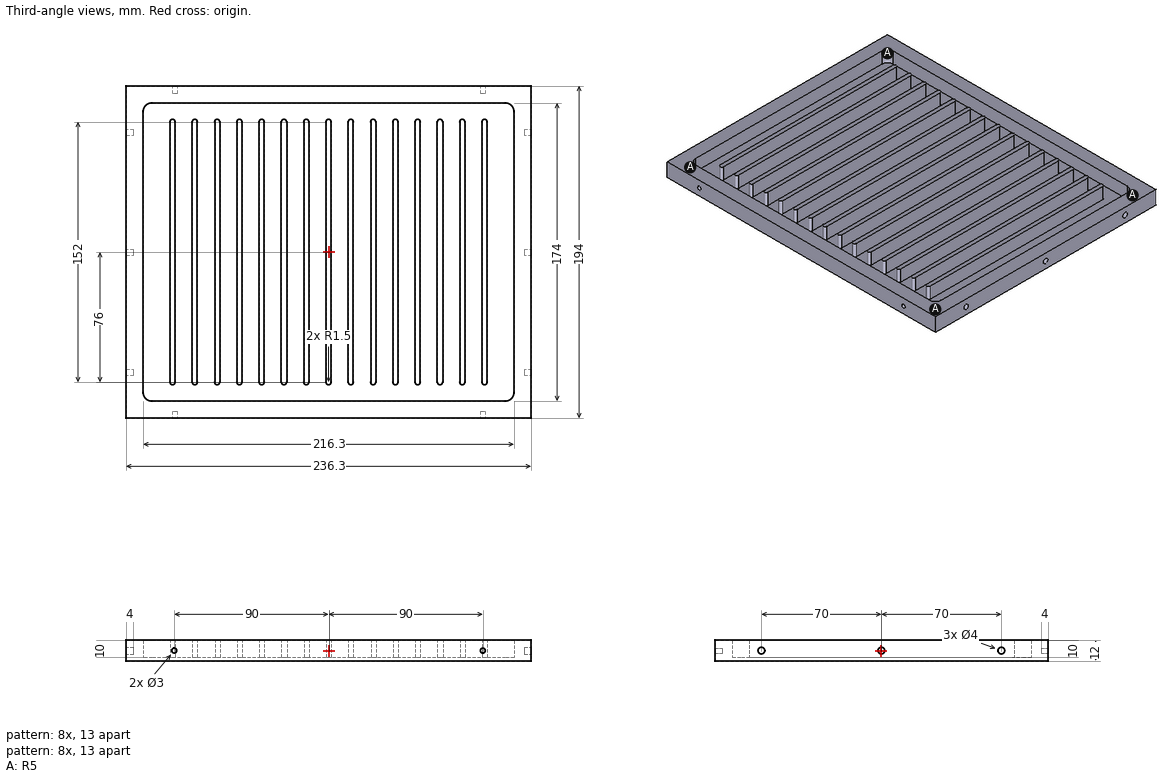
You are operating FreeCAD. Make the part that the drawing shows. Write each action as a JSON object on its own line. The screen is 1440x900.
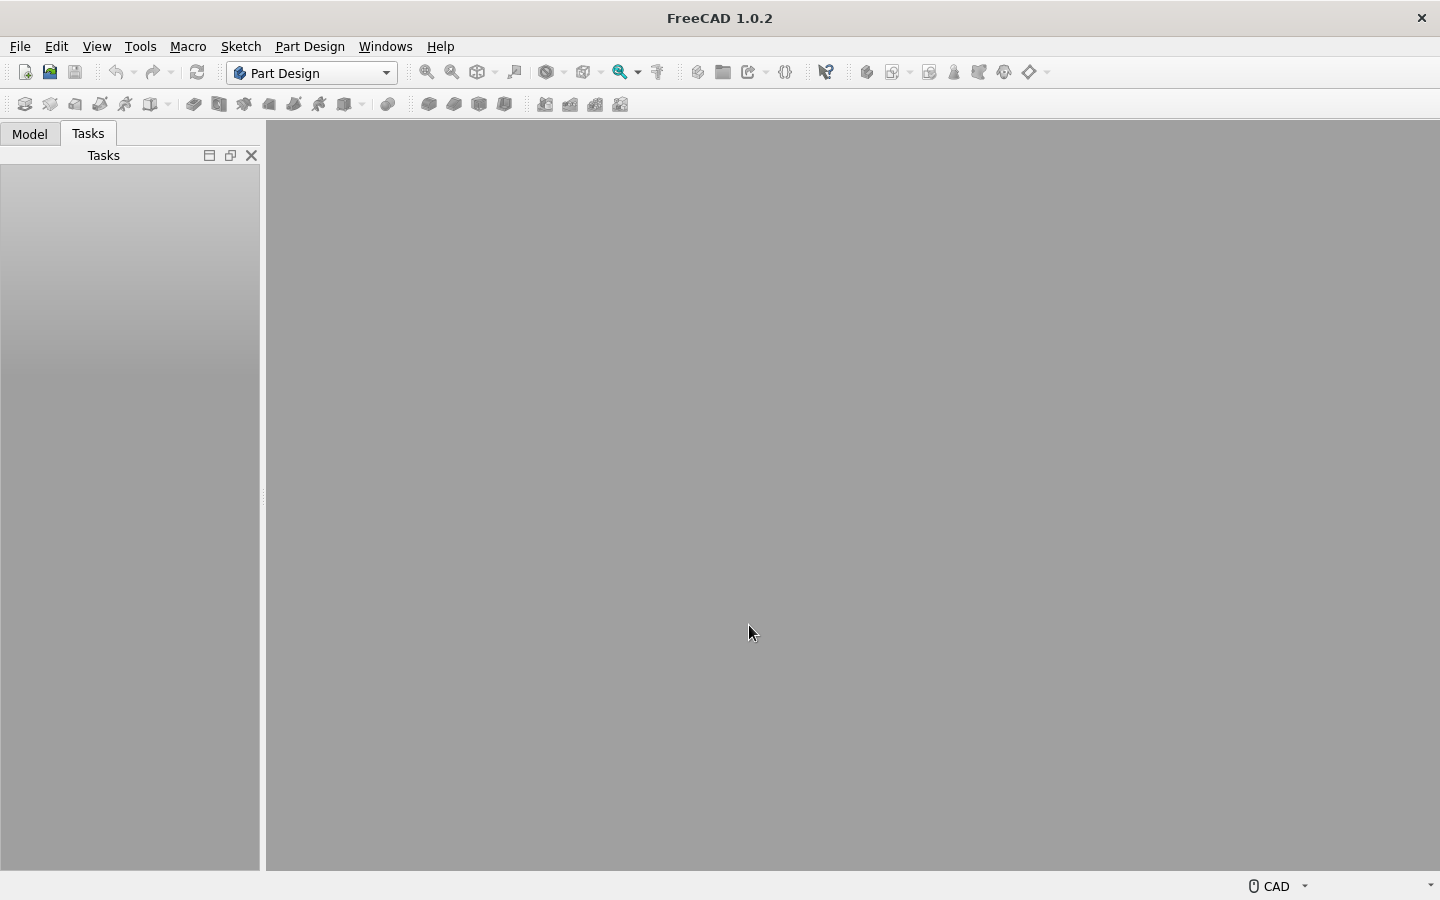
{"action": "left_click", "coordinate": [25, 72]}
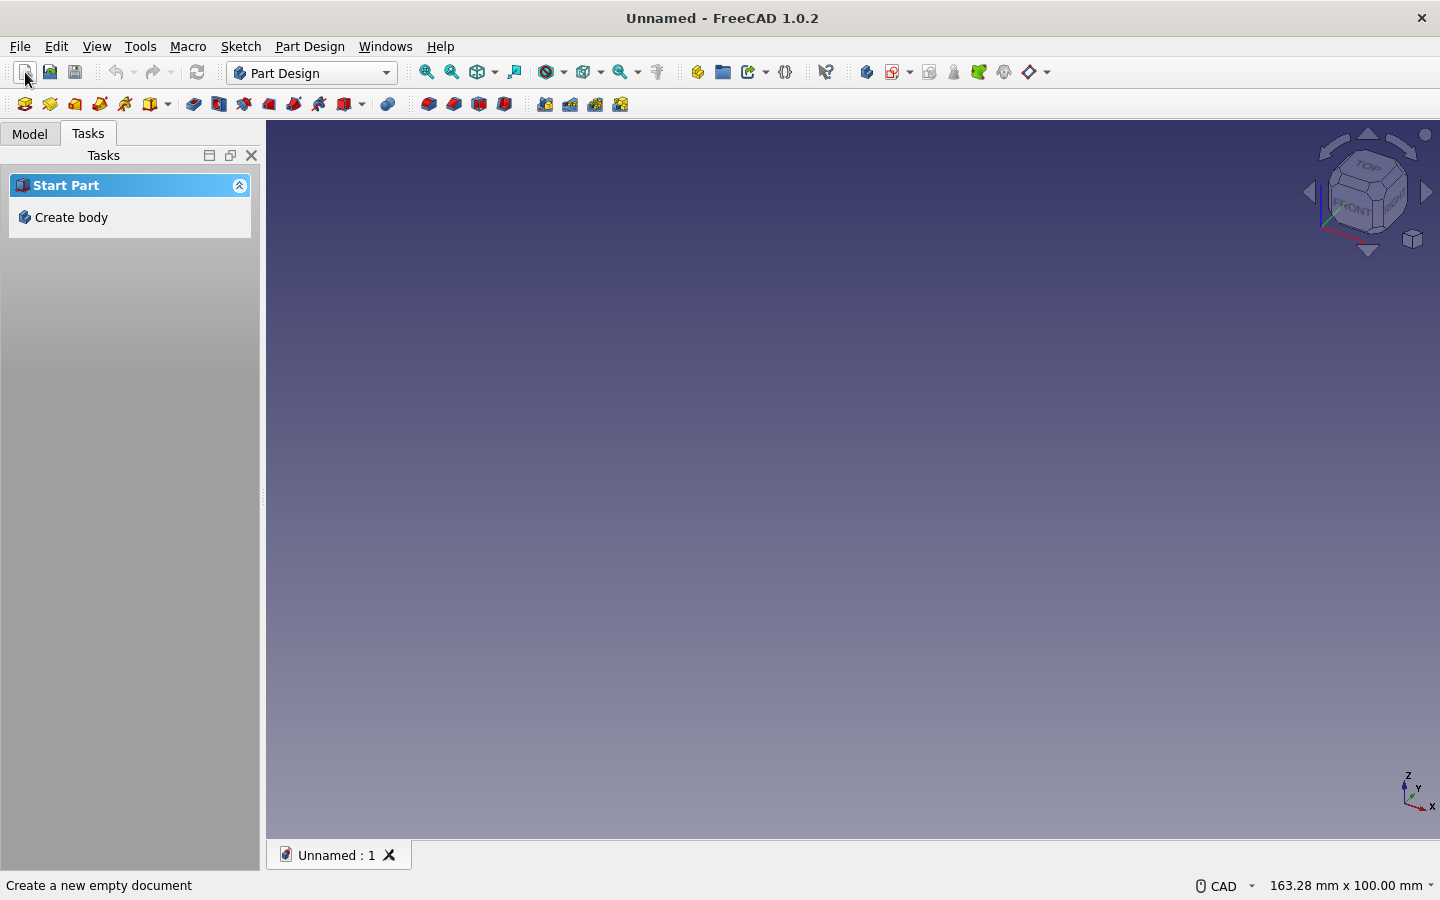
{"action": "left_click", "coordinate": [892, 72]}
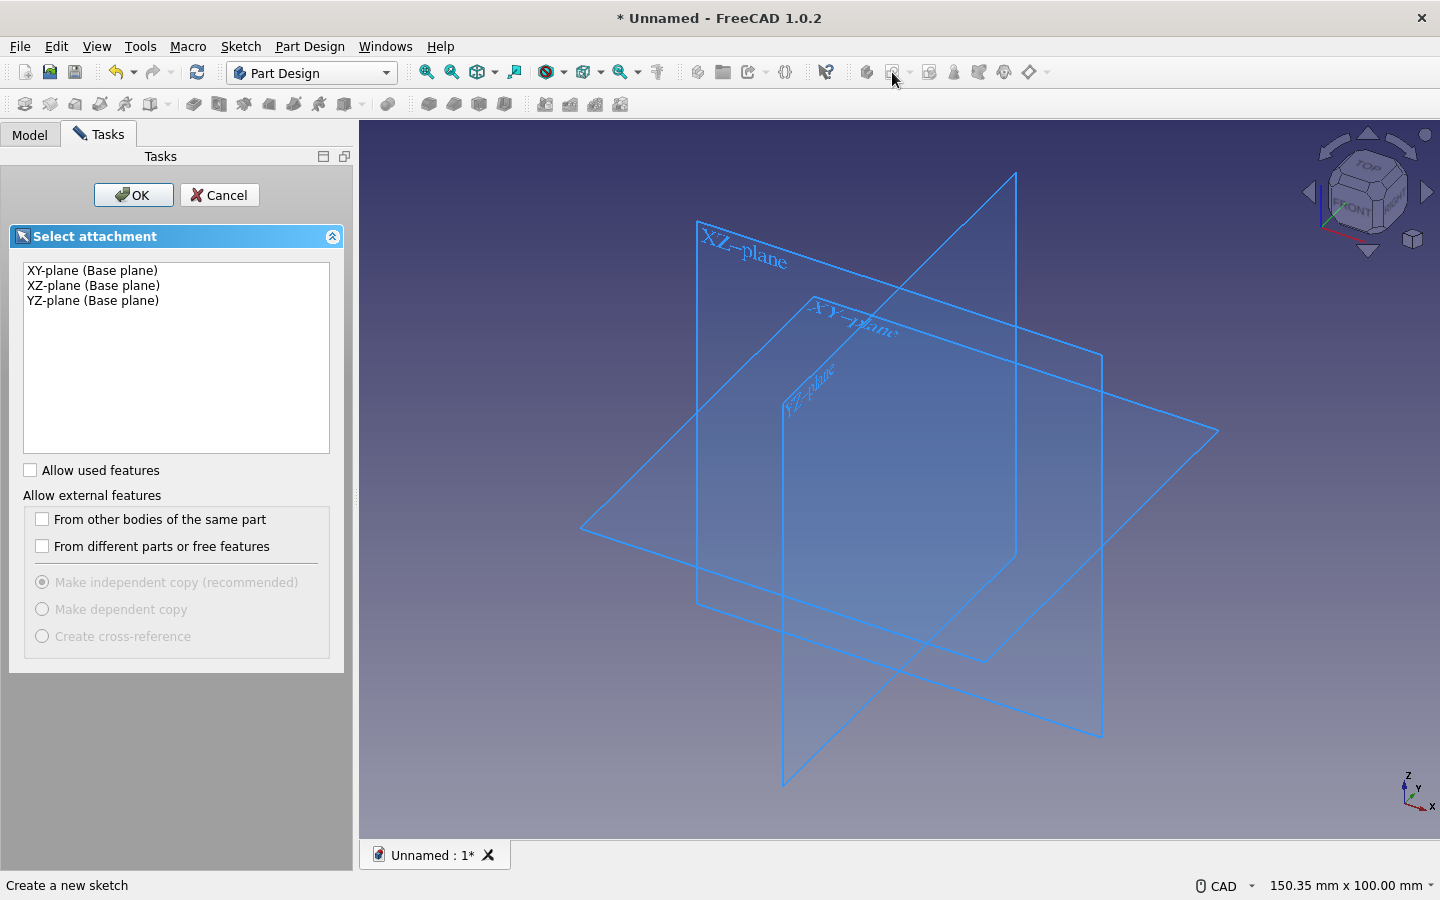
{"action": "left_click", "coordinate": [84, 270]}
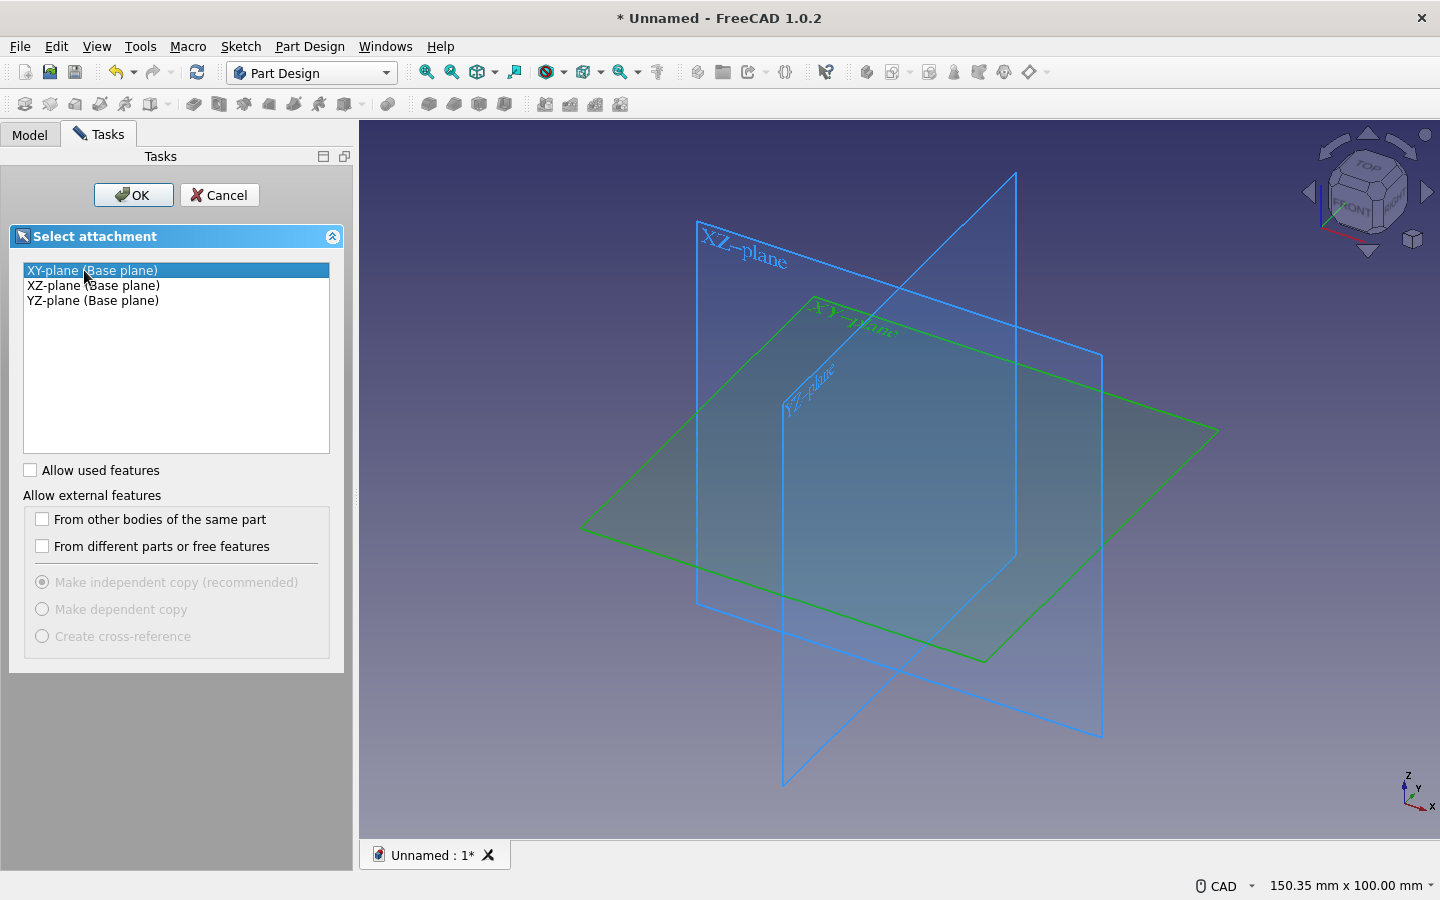
{"action": "left_click", "coordinate": [134, 195]}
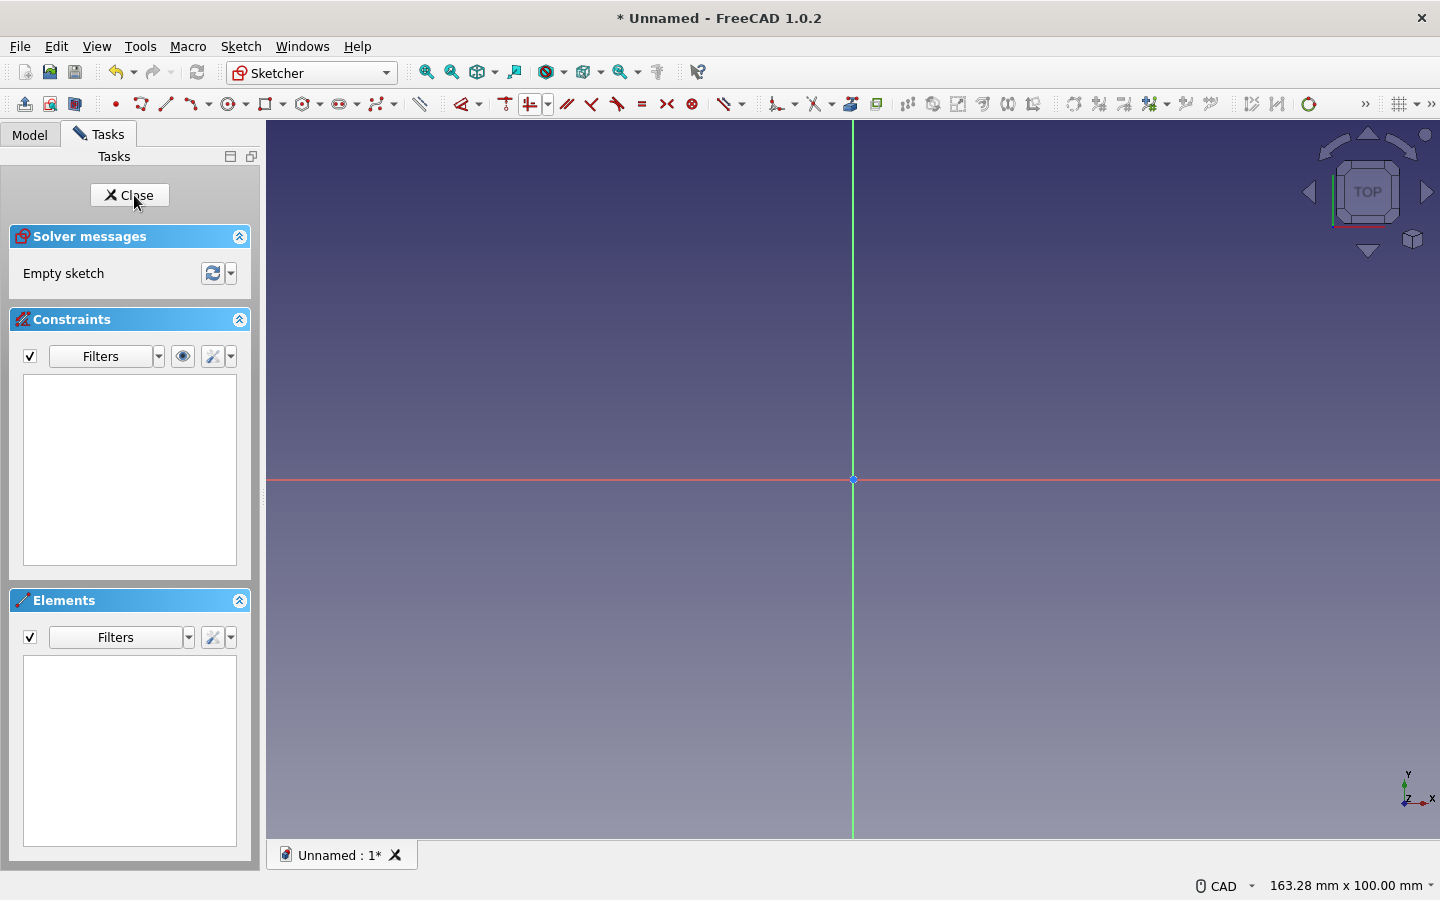
{"action": "scroll", "coordinate": [745, 480], "scroll_direction": "down", "scroll_amount": 5}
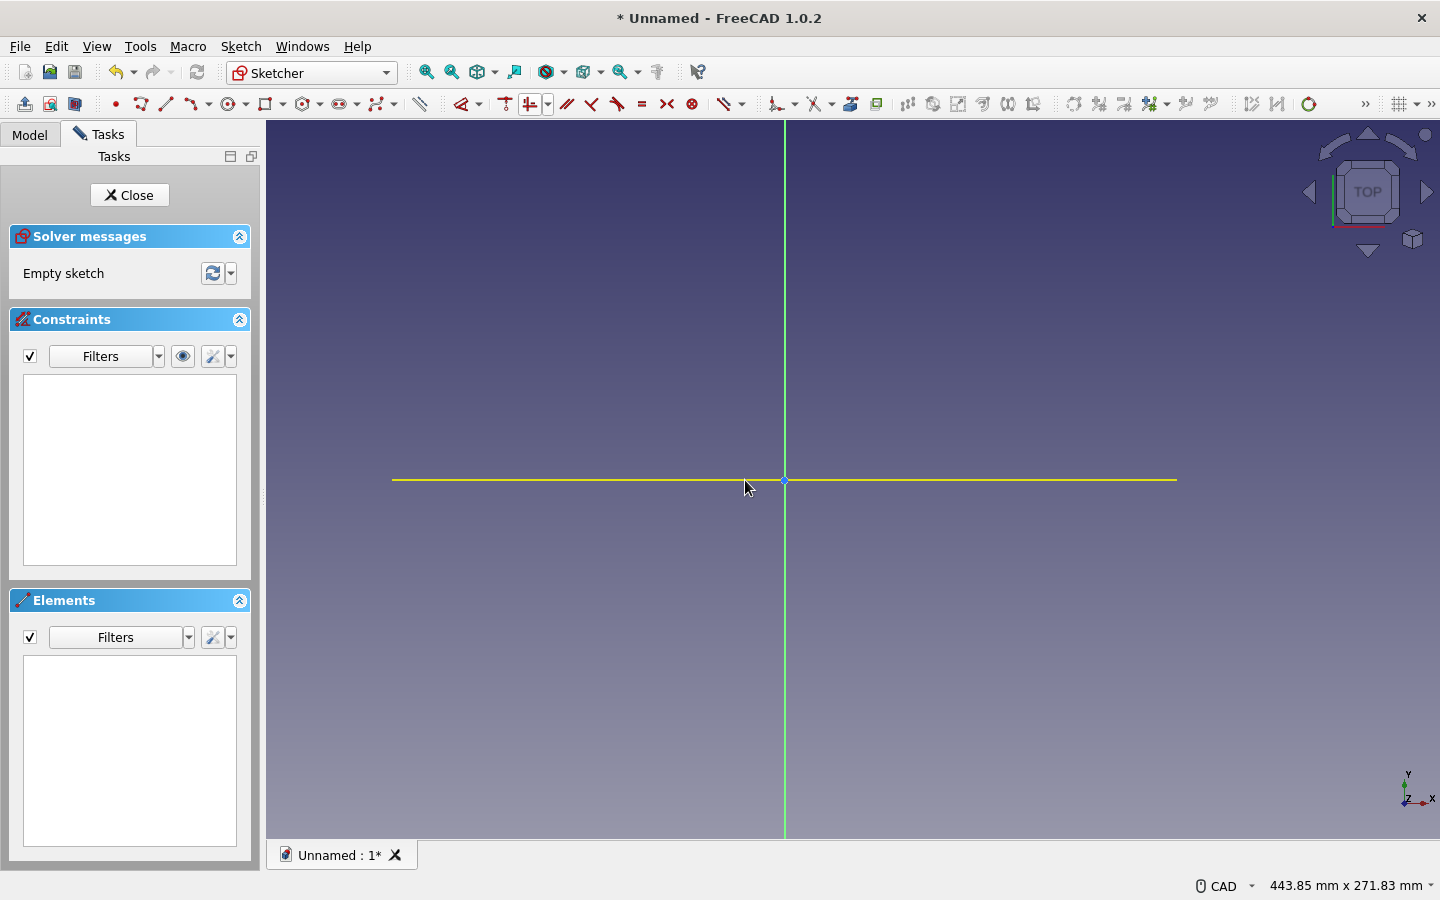
{"action": "key", "text": "g v"}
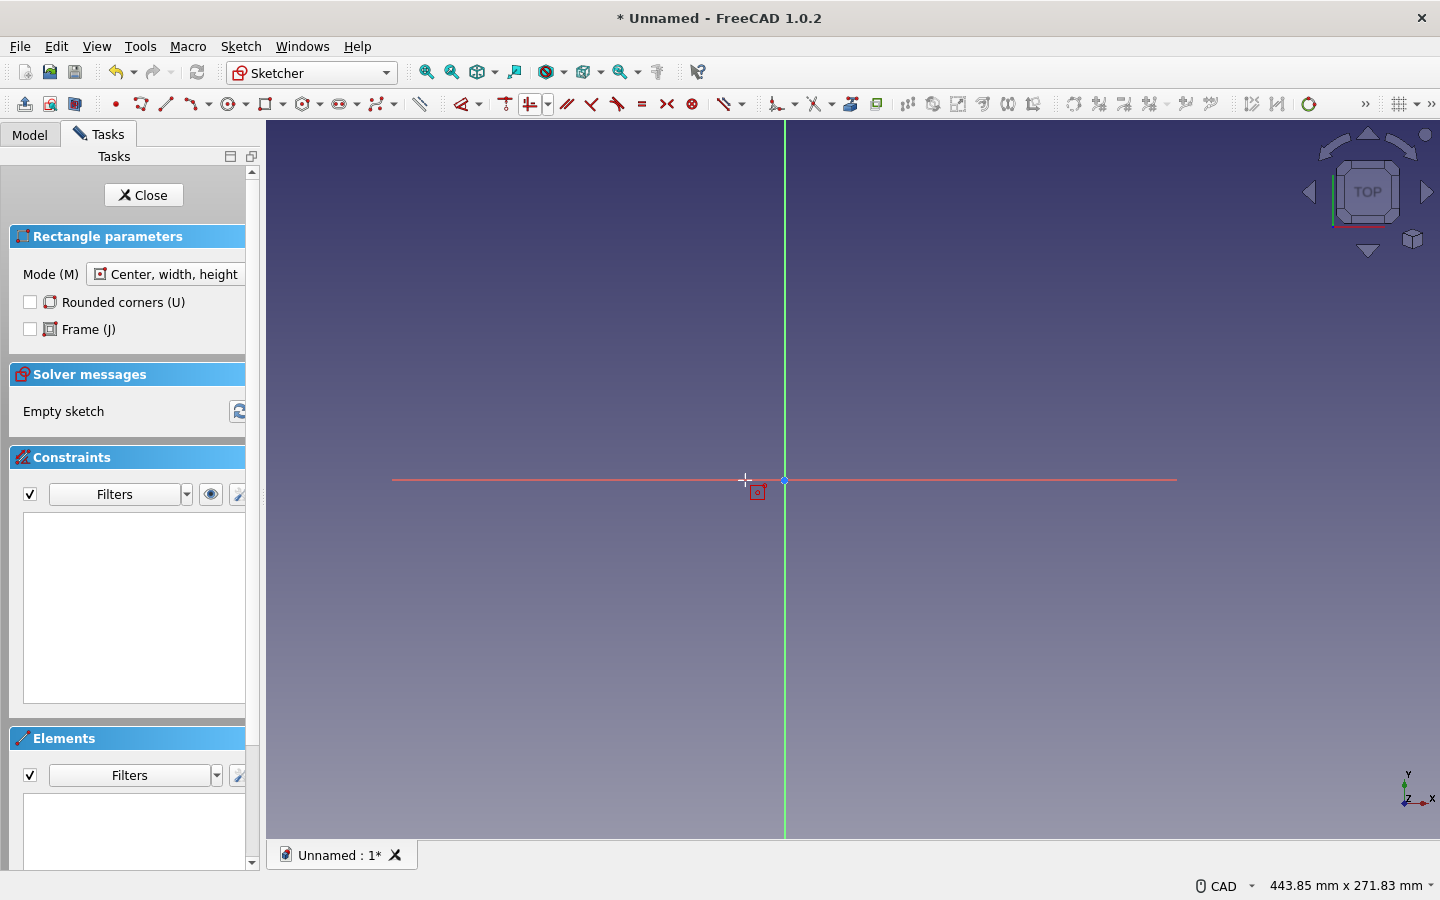
{"action": "left_click", "coordinate": [785, 480]}
{"action": "left_click", "coordinate": [1098, 224]}
{"action": "key", "text": "Escape"}